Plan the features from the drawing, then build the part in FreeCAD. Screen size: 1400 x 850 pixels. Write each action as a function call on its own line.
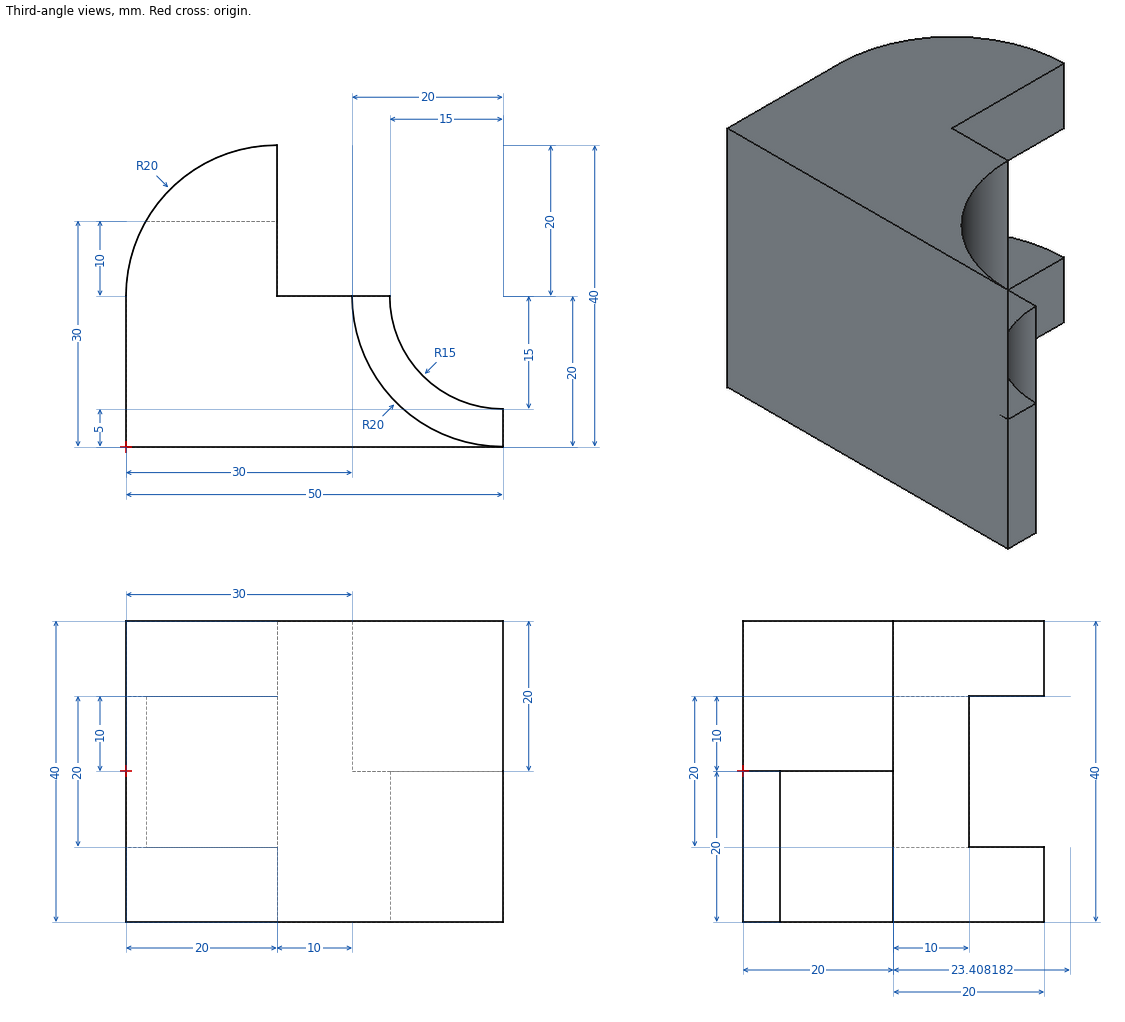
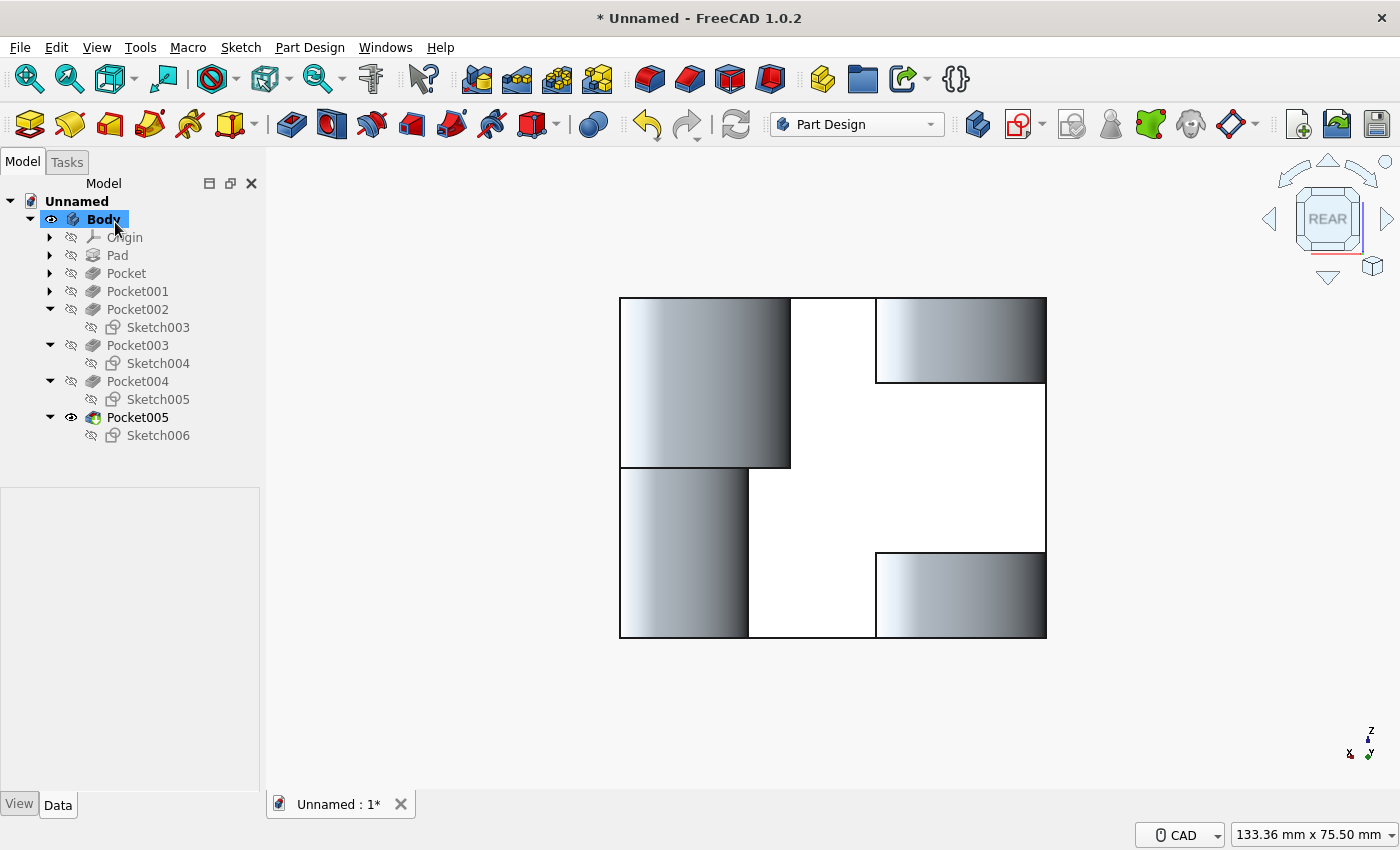
click(897, 467)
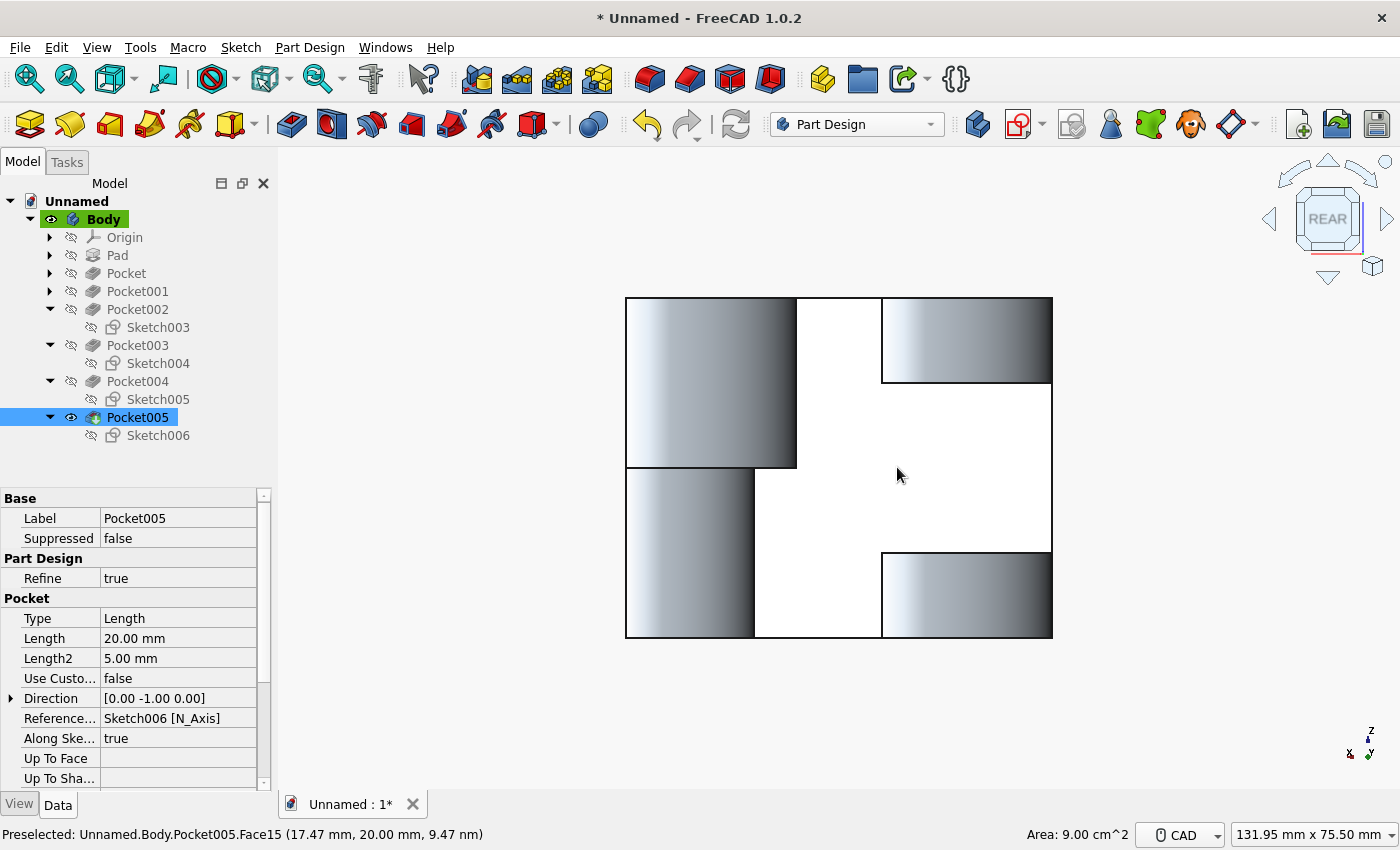
click(1018, 124)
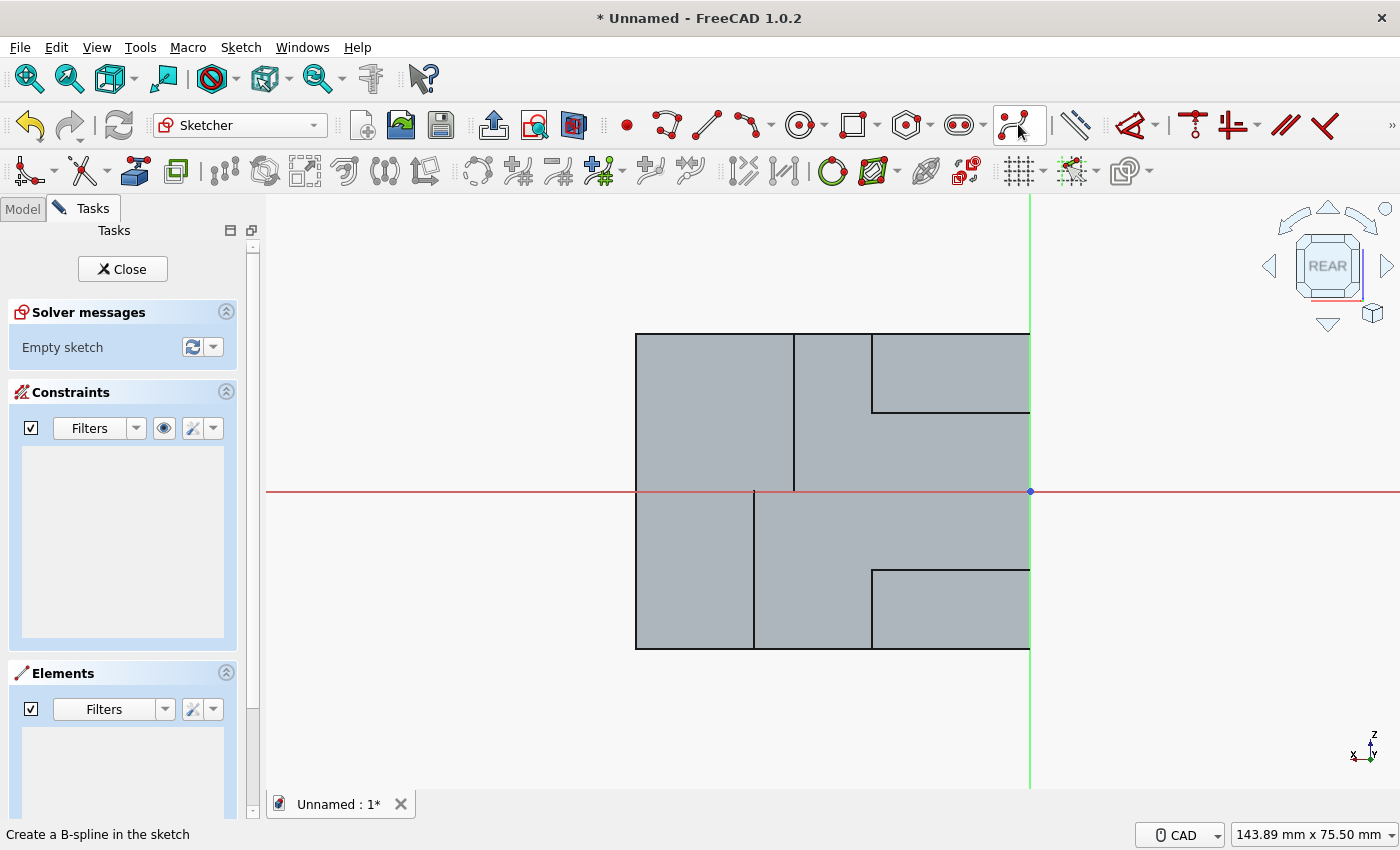
click(574, 126)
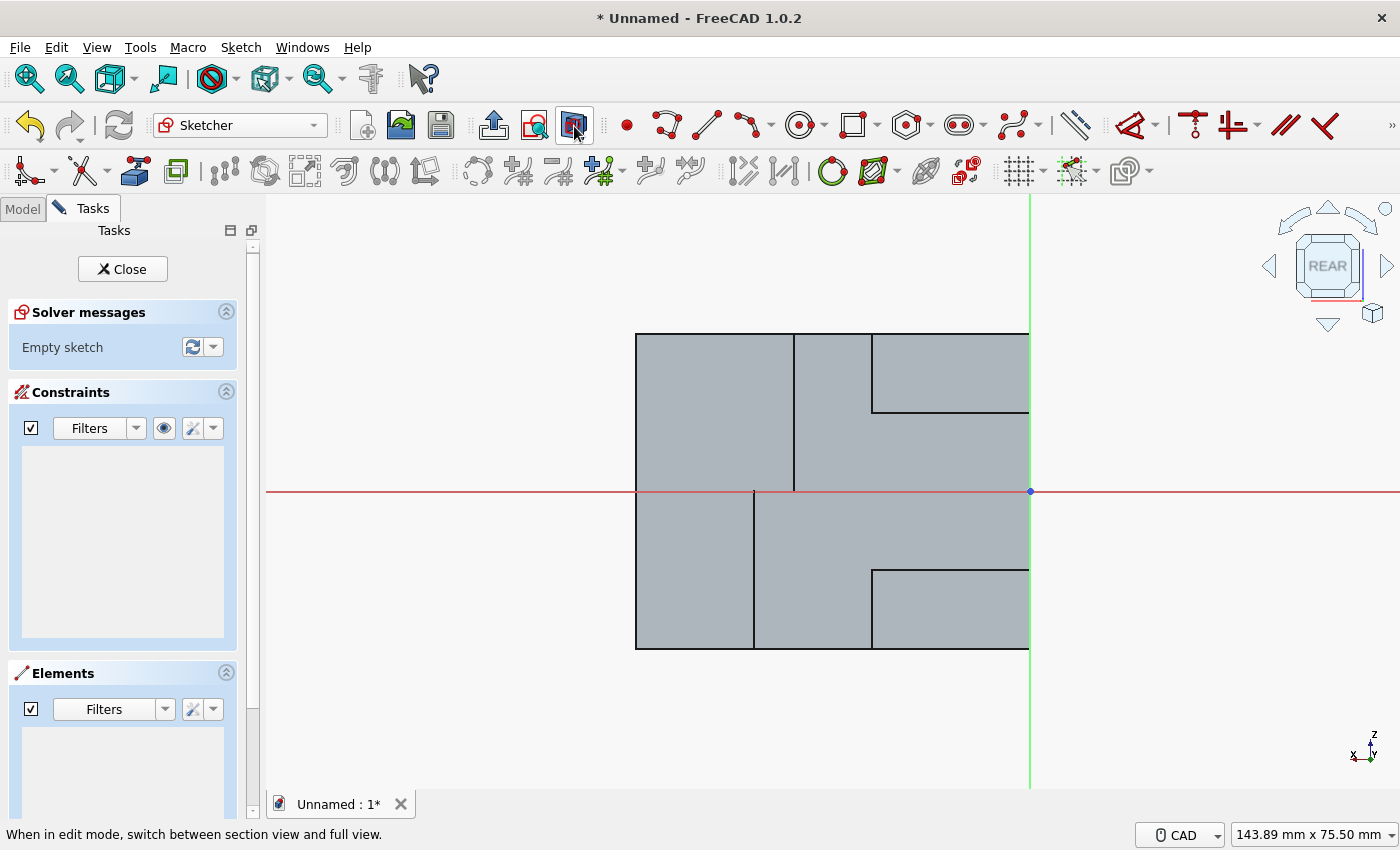
scroll(1104, 492, up, 4)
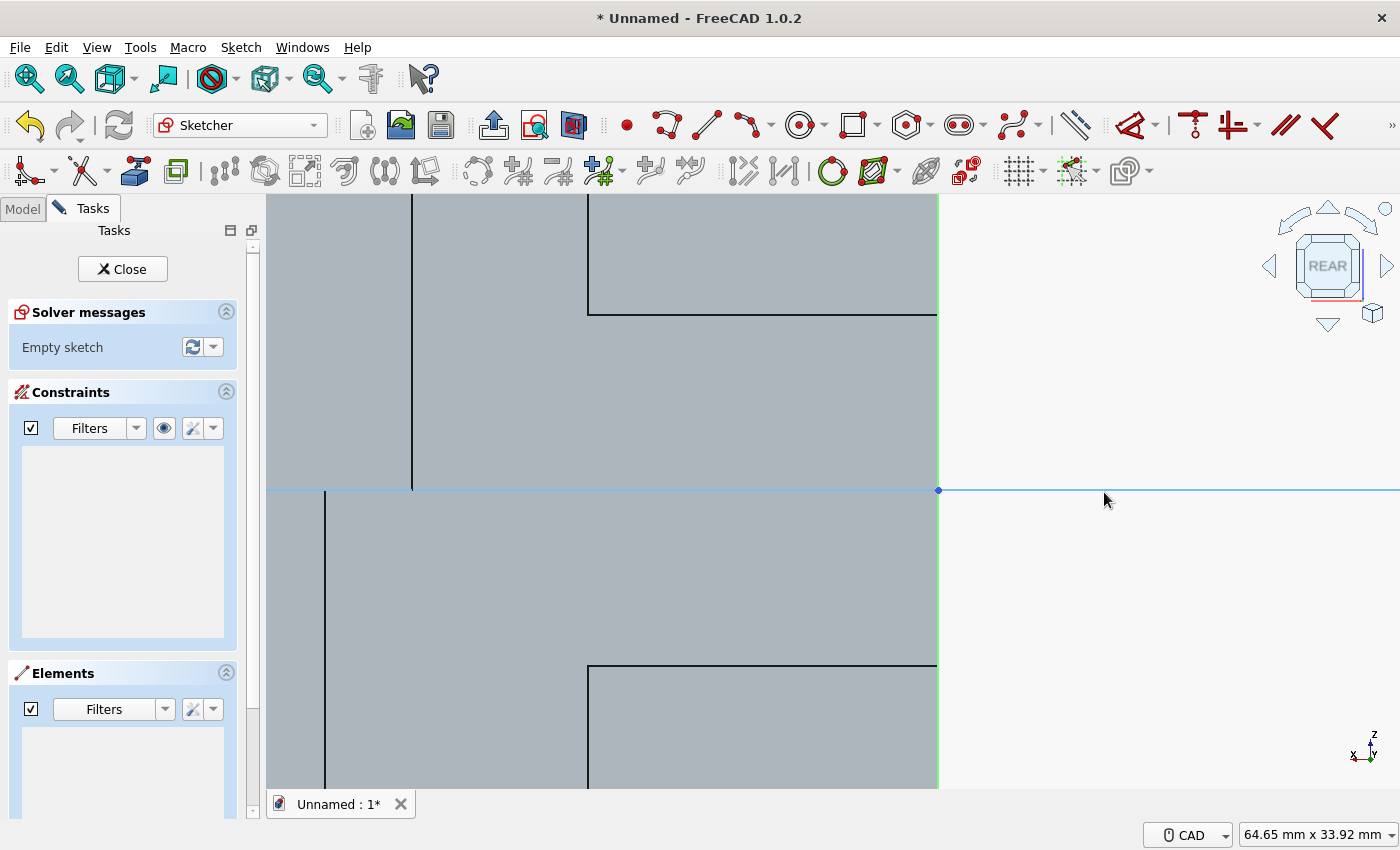
key(g)
key(r)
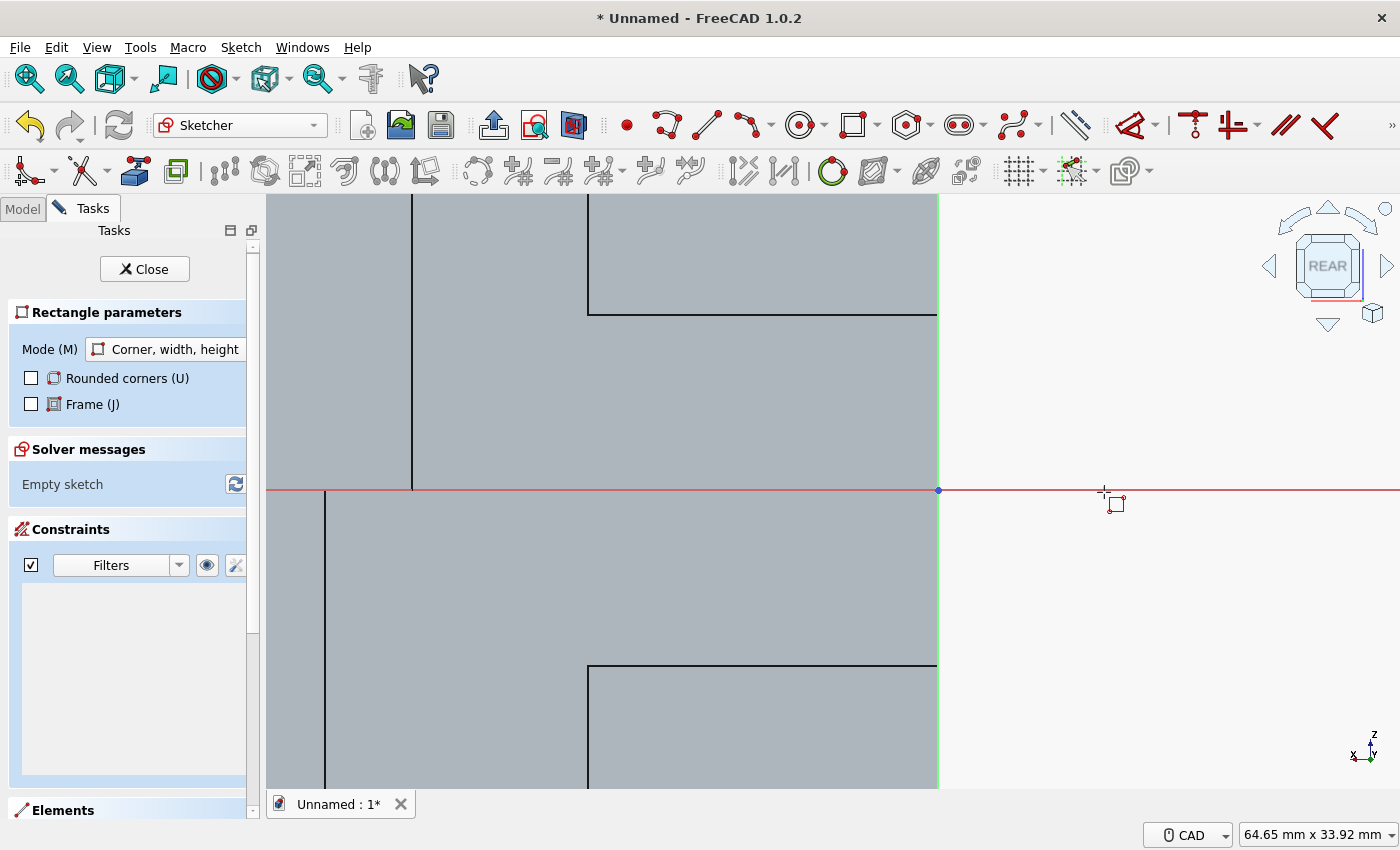
click(588, 315)
click(938, 666)
key(Escape)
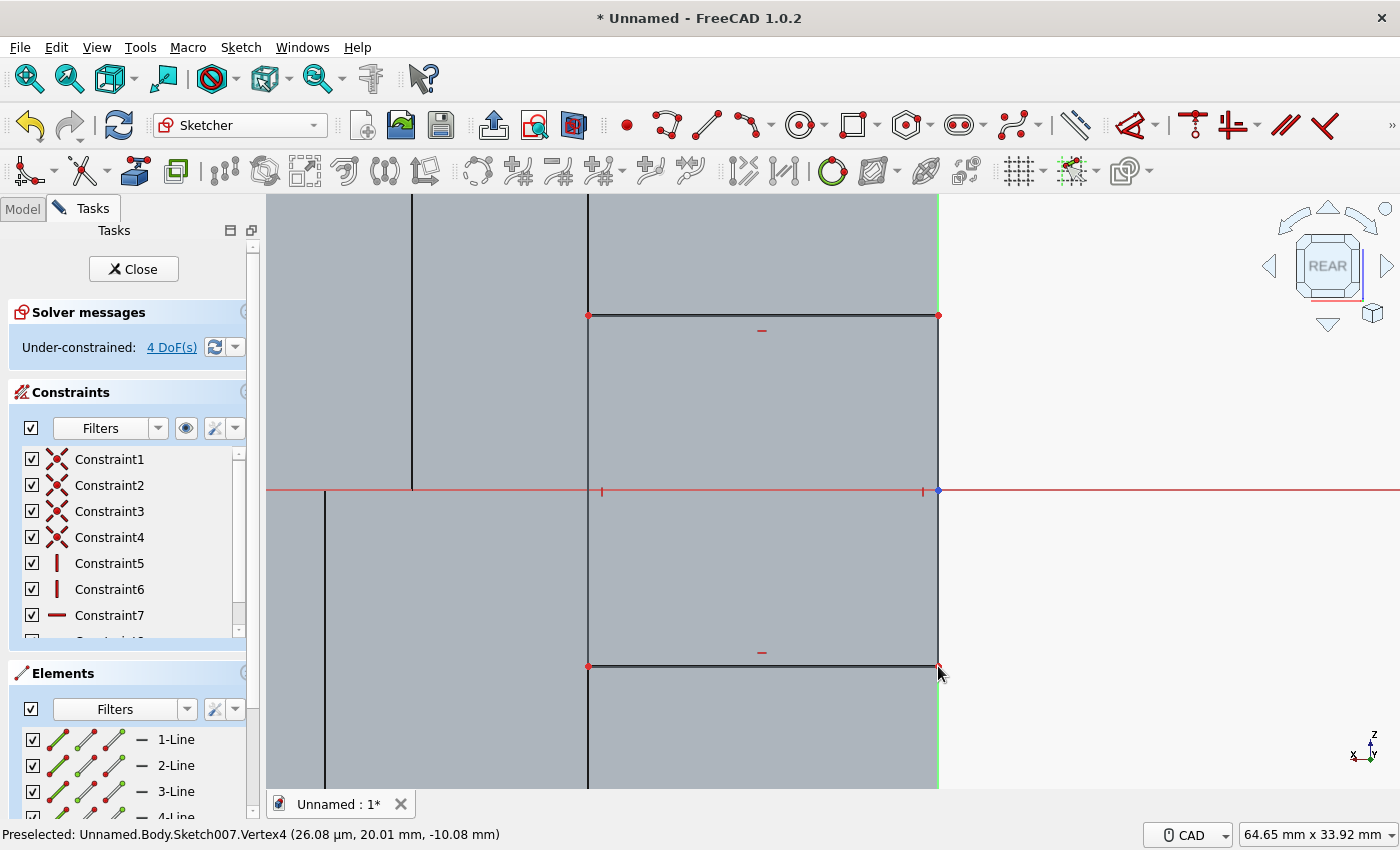
click(938, 667)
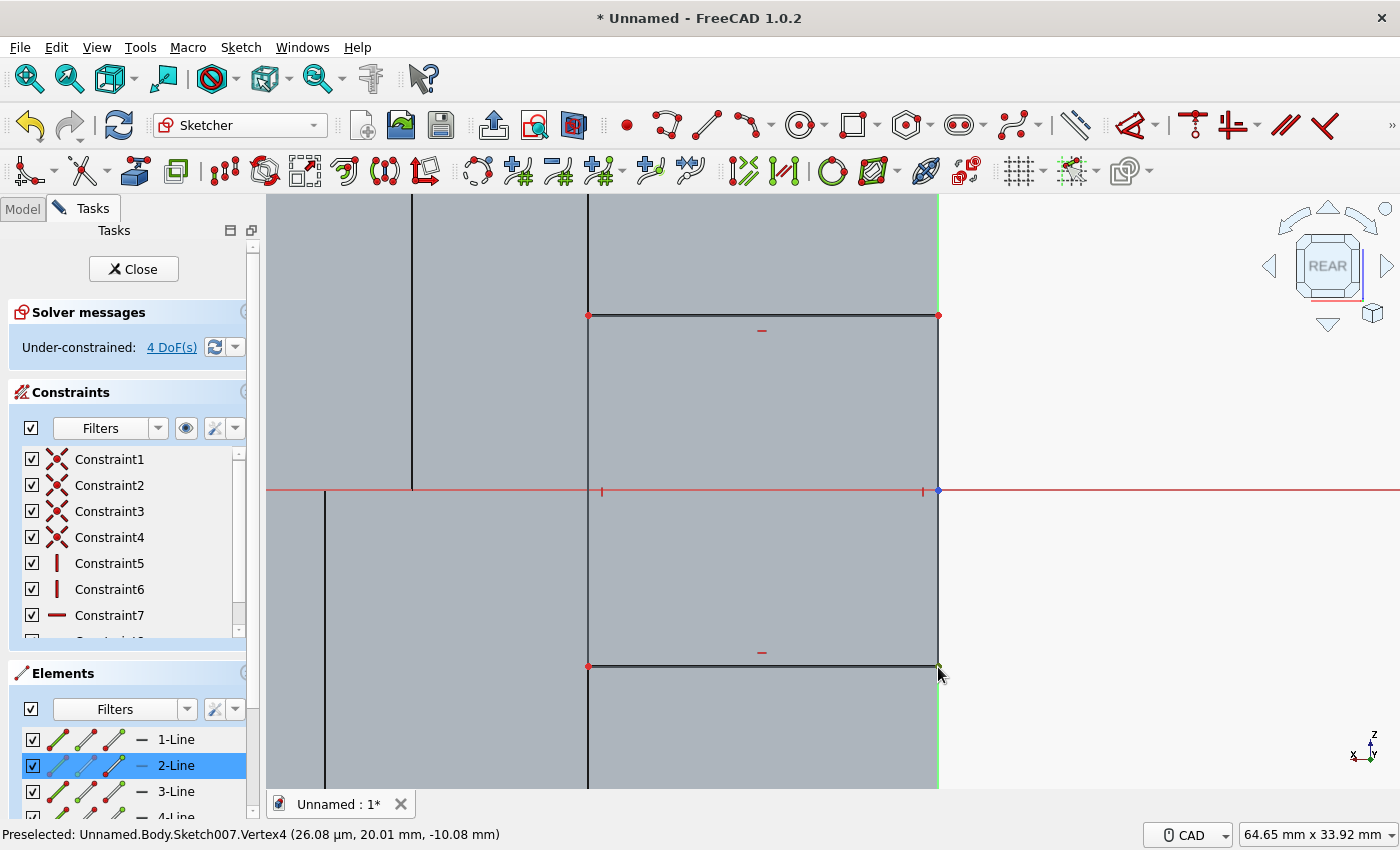
click(938, 722)